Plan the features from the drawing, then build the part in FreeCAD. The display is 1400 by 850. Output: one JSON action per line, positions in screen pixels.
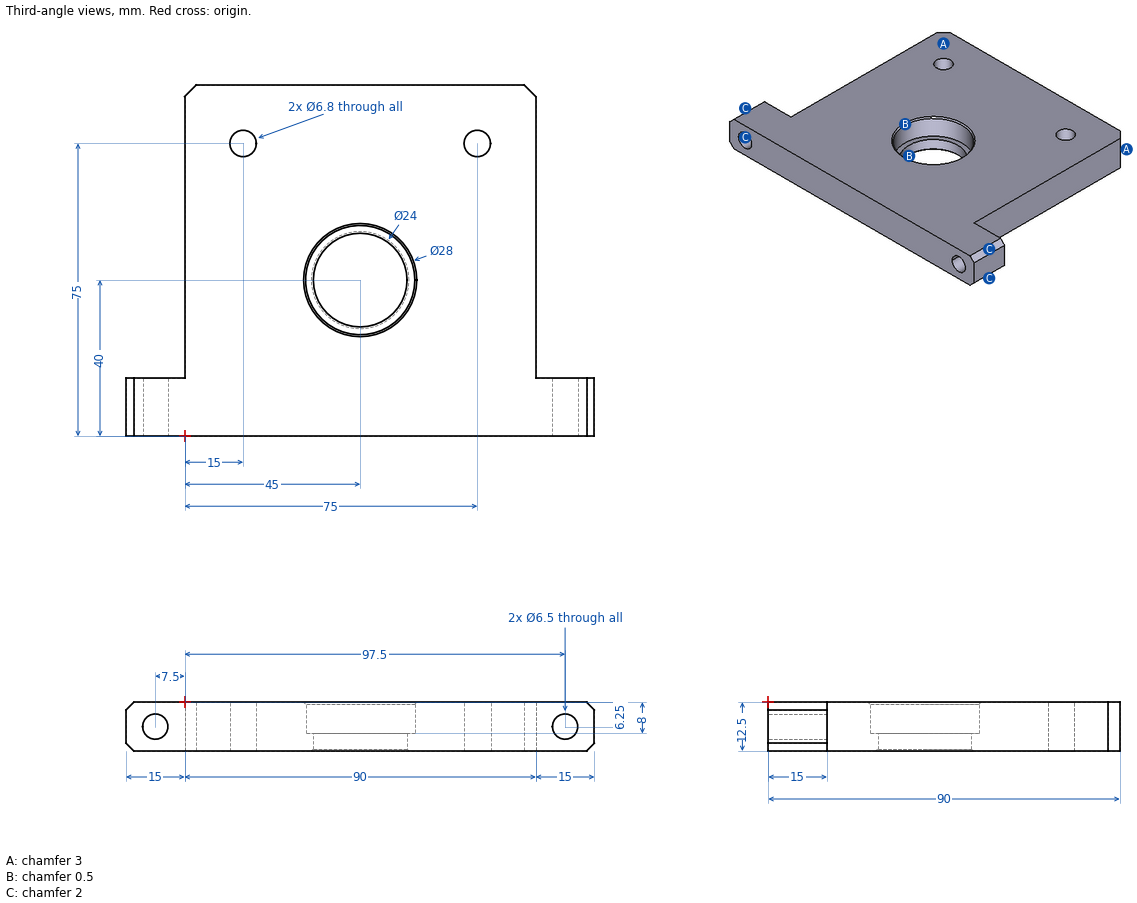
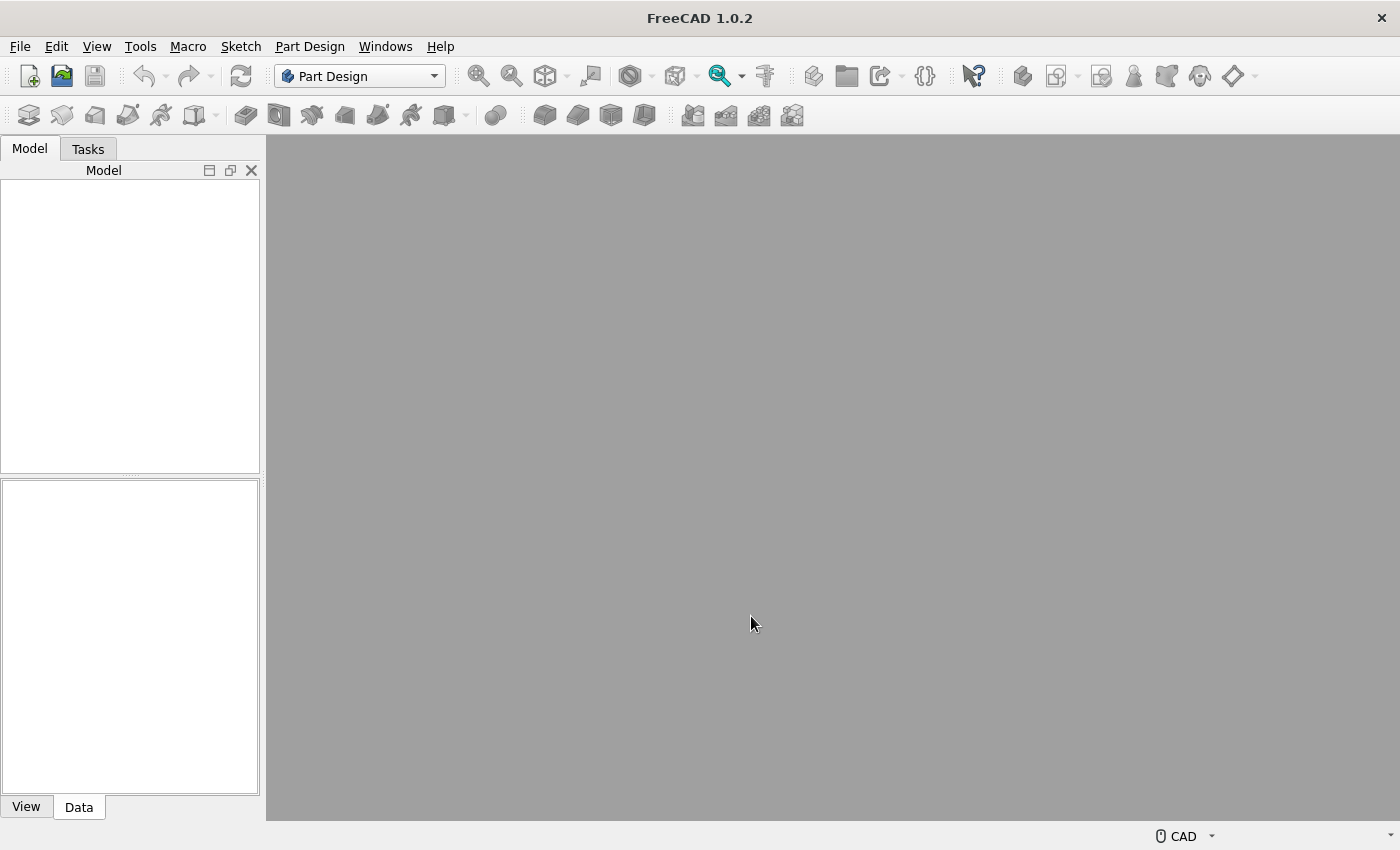
{"action": "left_click", "coordinate": [29, 76]}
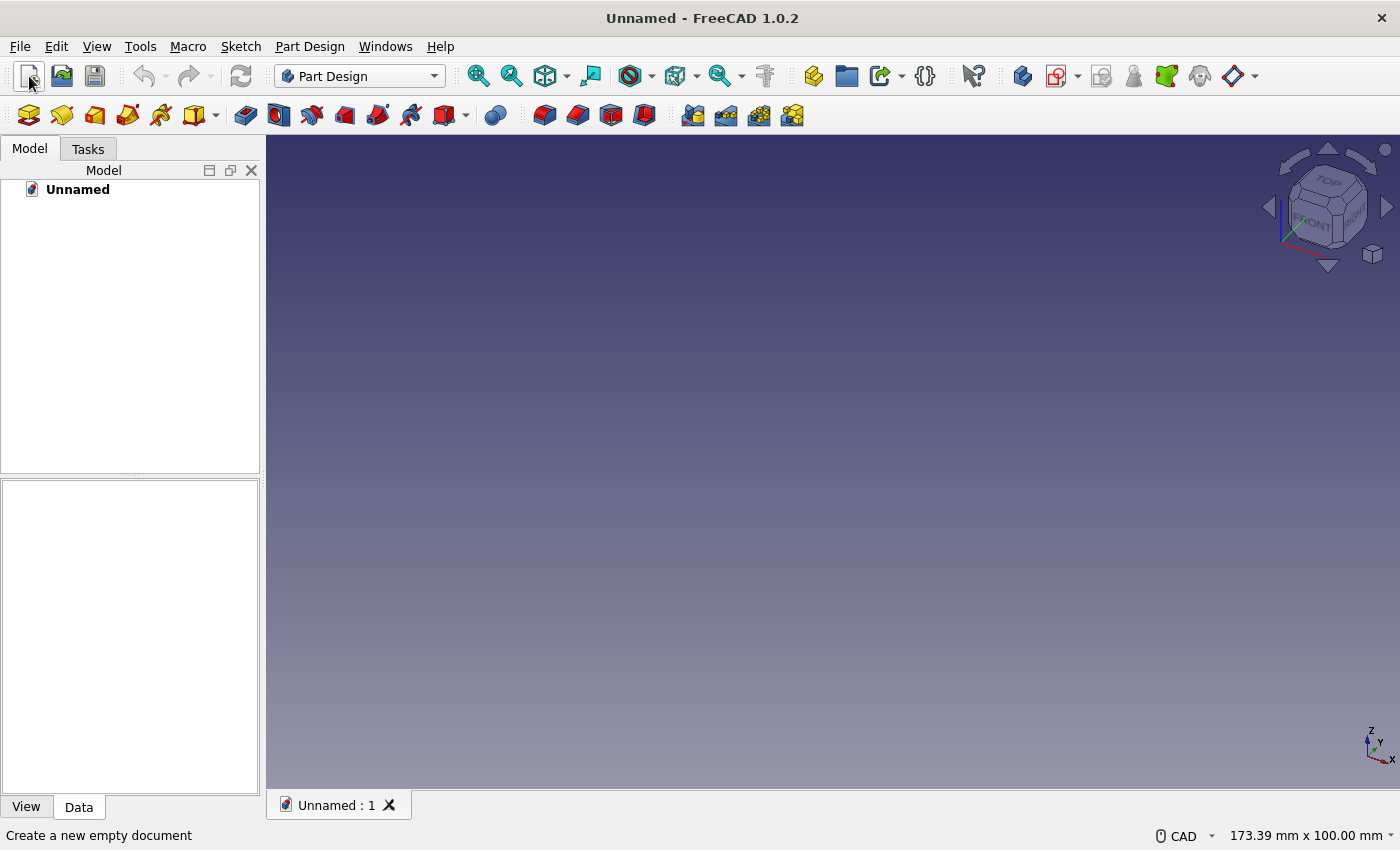
{"action": "left_click", "coordinate": [1056, 76]}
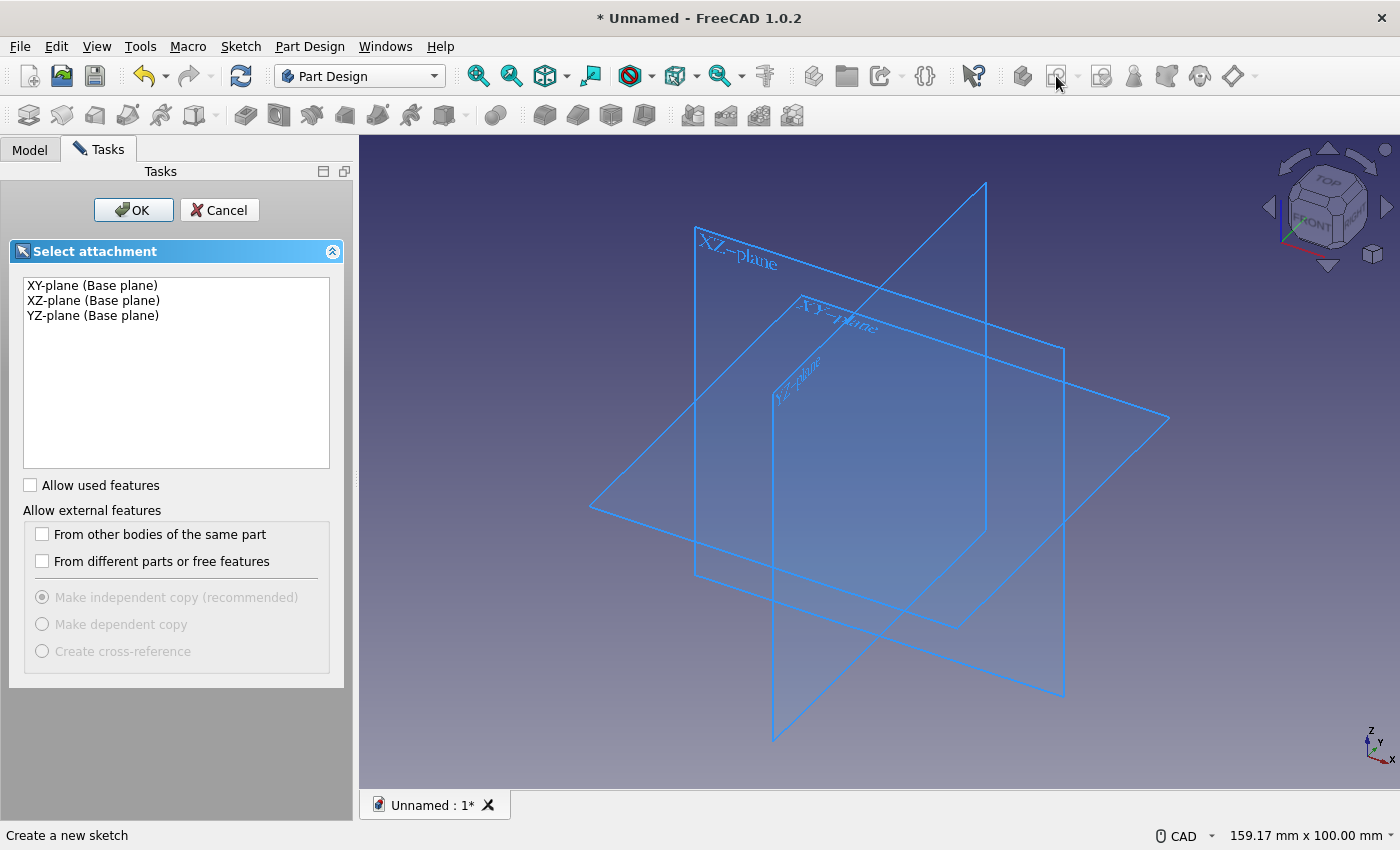
{"action": "left_click", "coordinate": [84, 316]}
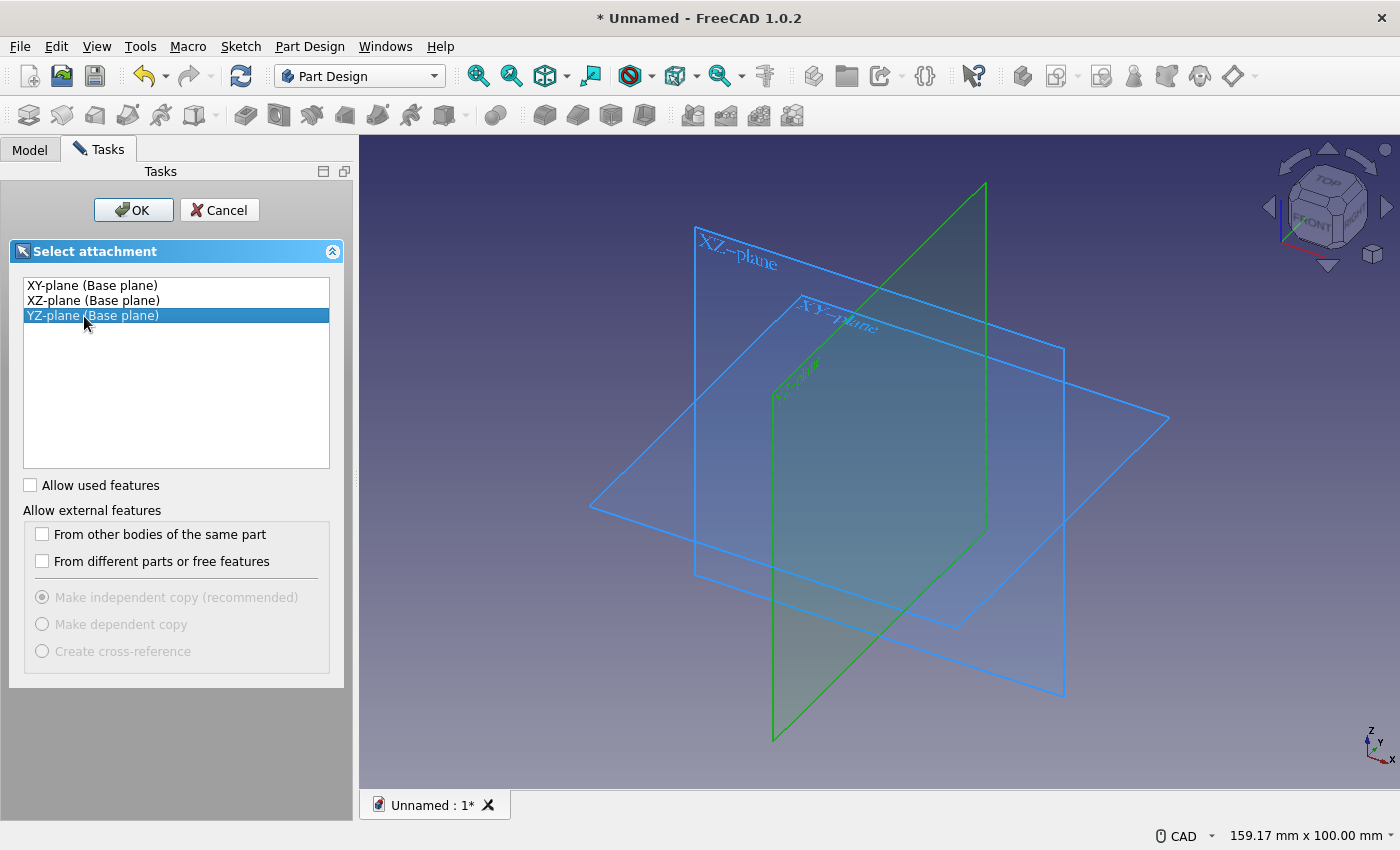
{"action": "left_click", "coordinate": [134, 210]}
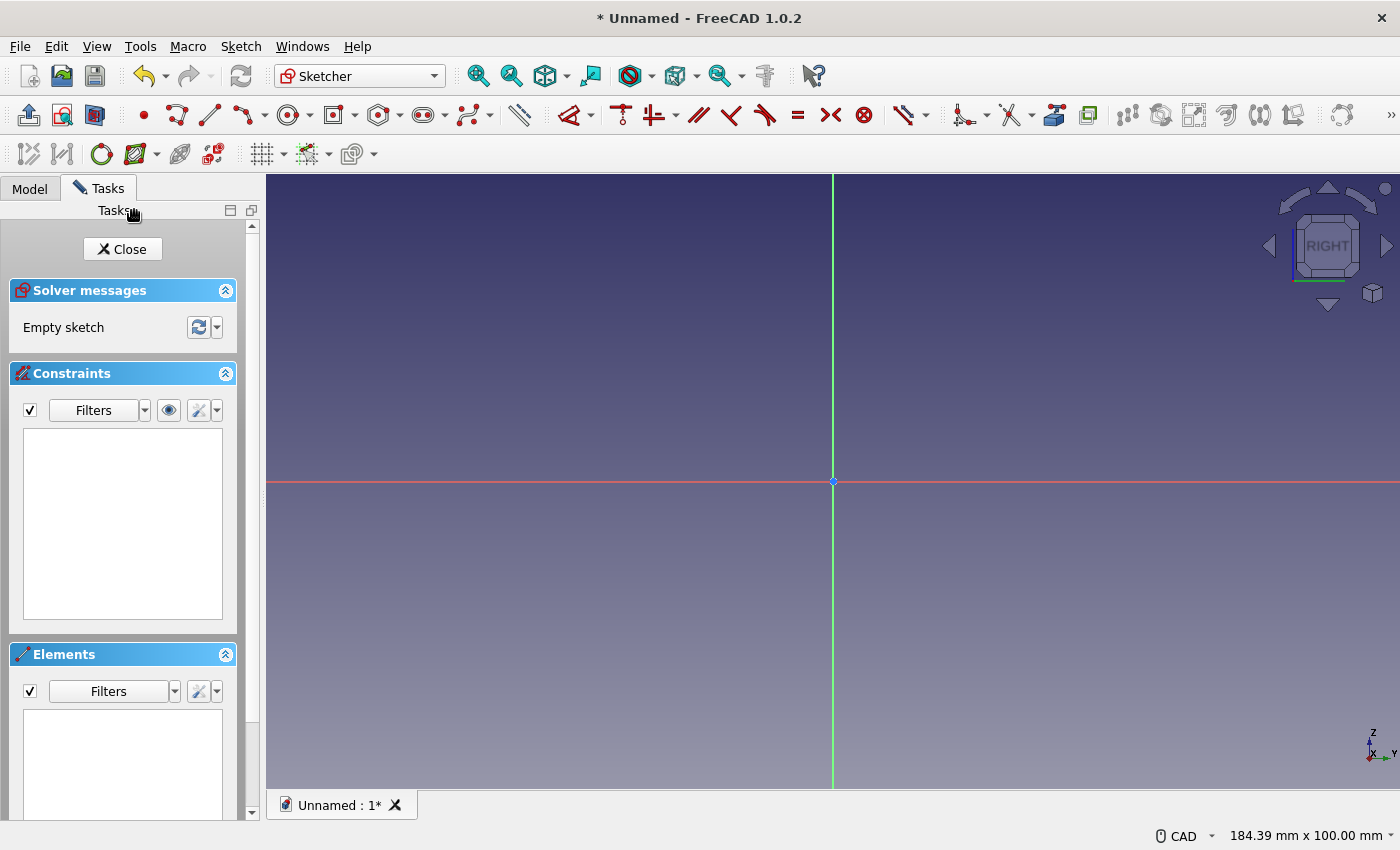
{"action": "scroll", "coordinate": [294, 308], "scroll_direction": "down", "scroll_amount": 1}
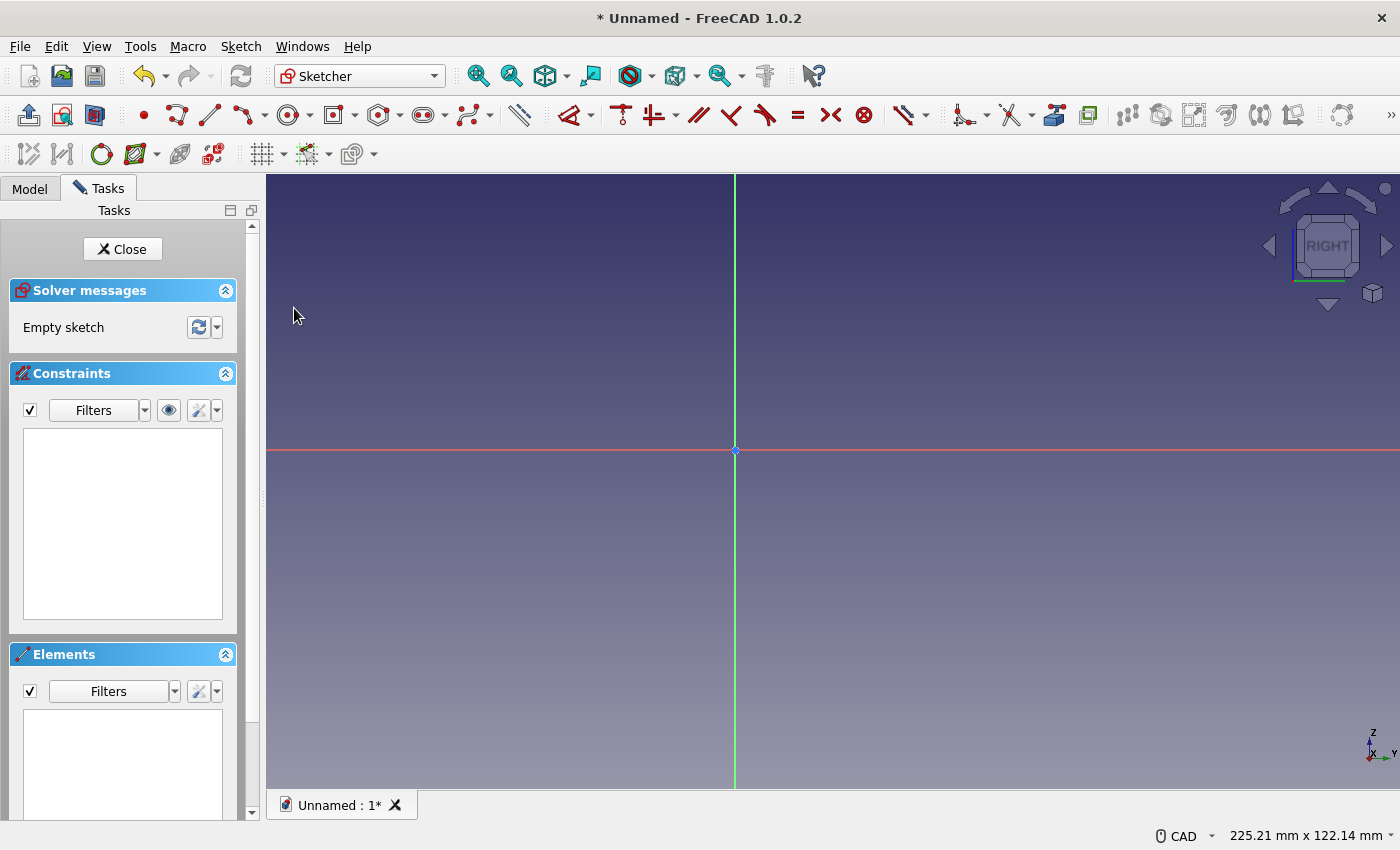
{"action": "scroll", "coordinate": [1235, 482], "scroll_direction": "up", "scroll_amount": 2}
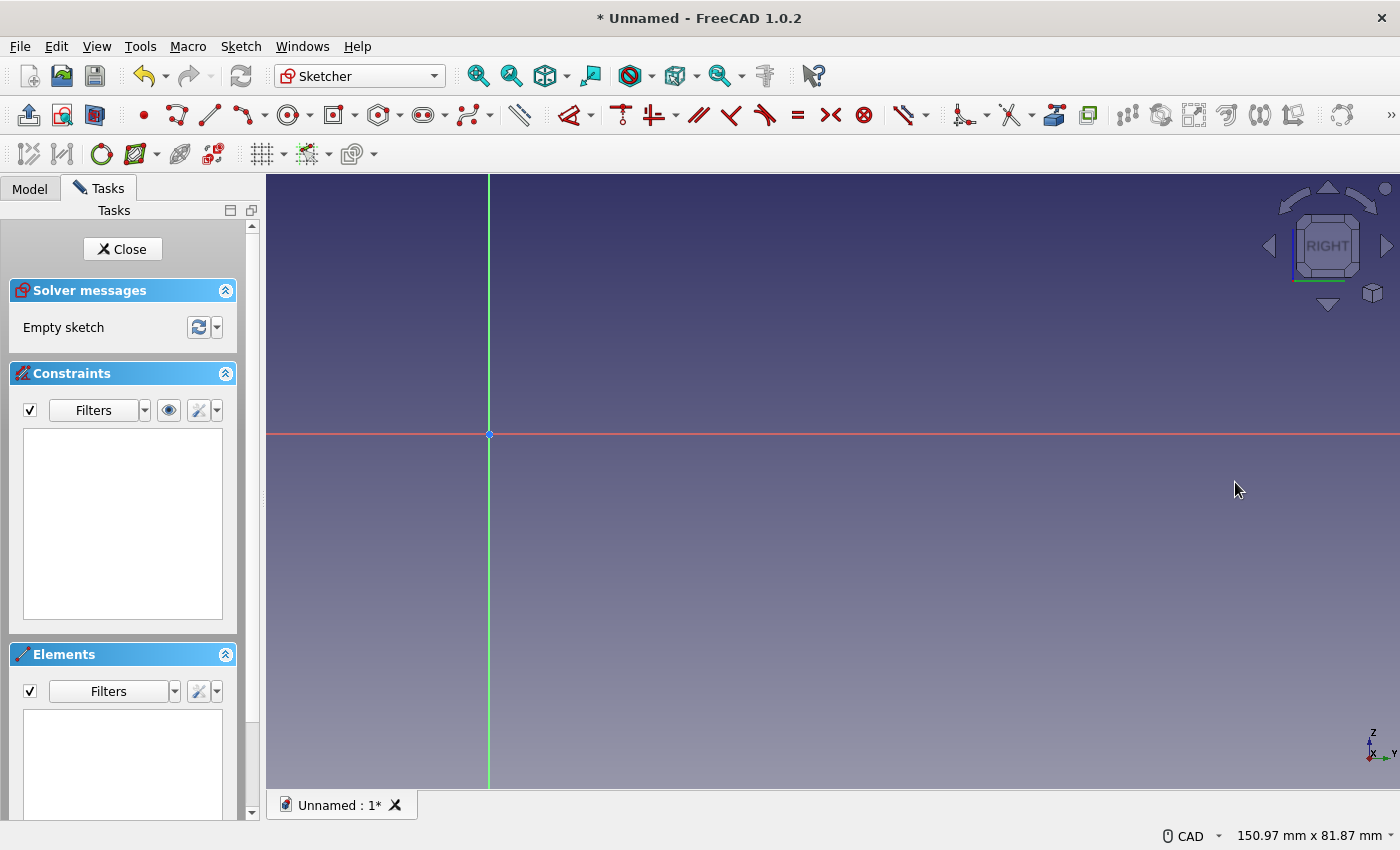
{"action": "left_click", "coordinate": [354, 116]}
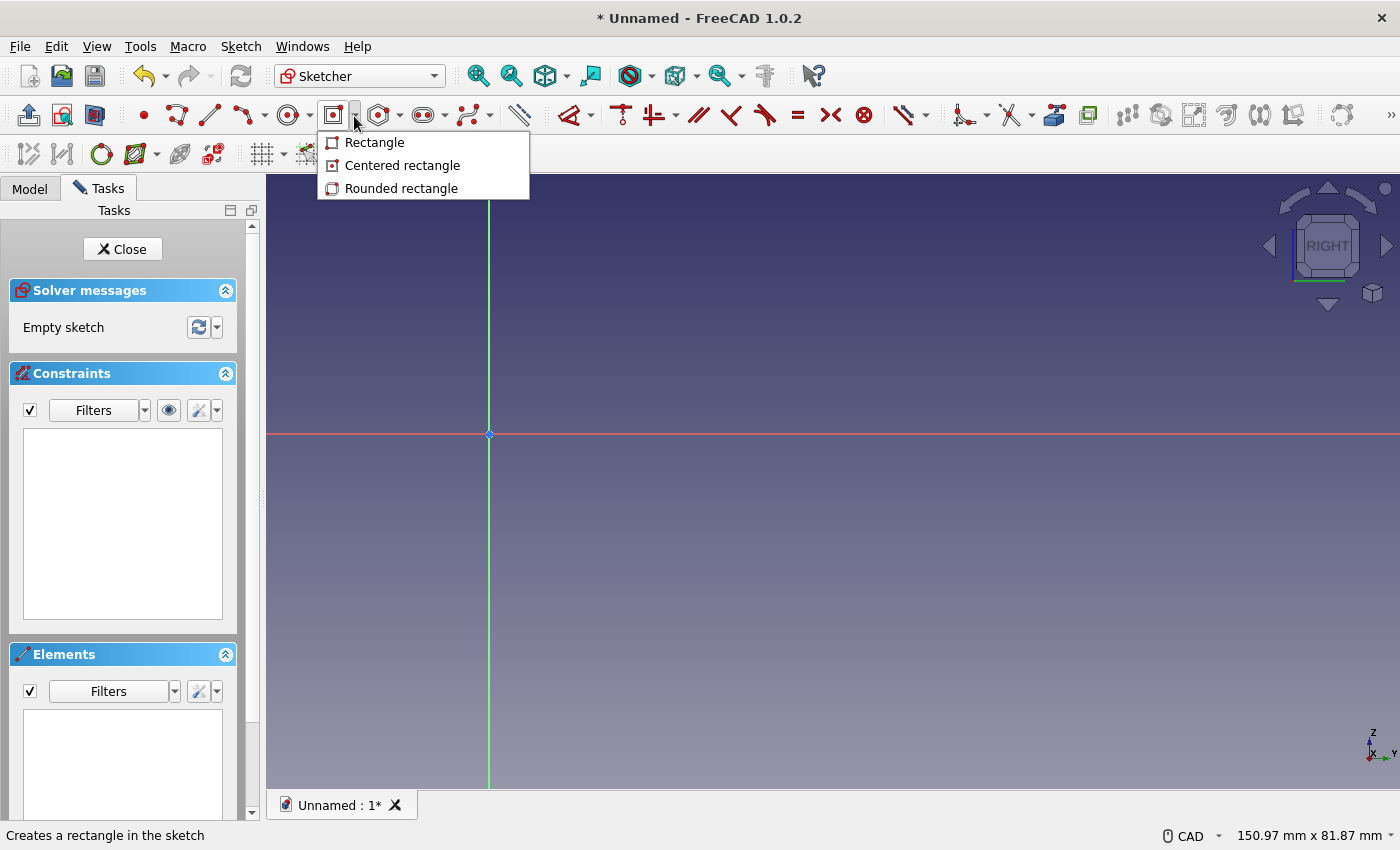
{"action": "left_click", "coordinate": [424, 142]}